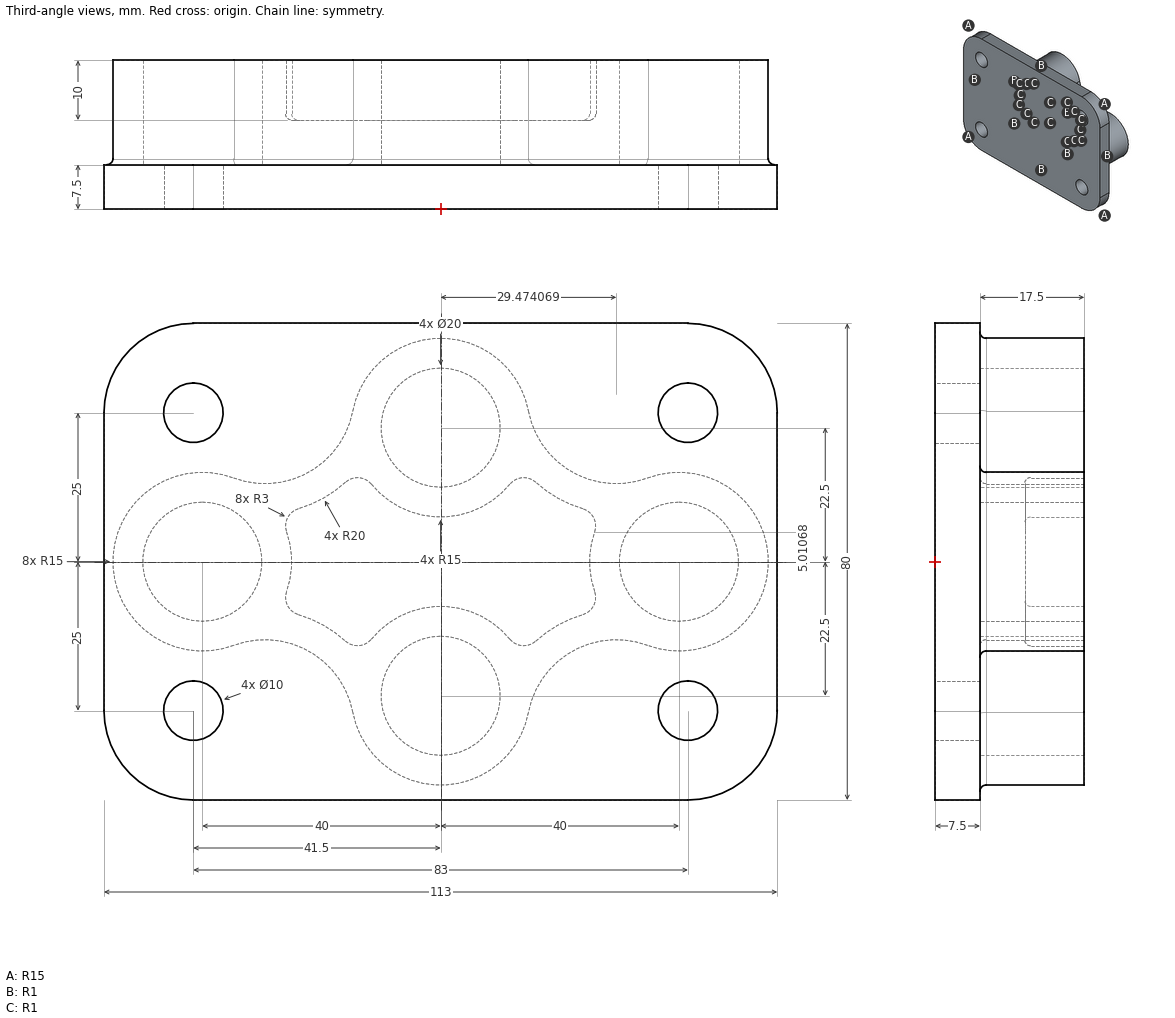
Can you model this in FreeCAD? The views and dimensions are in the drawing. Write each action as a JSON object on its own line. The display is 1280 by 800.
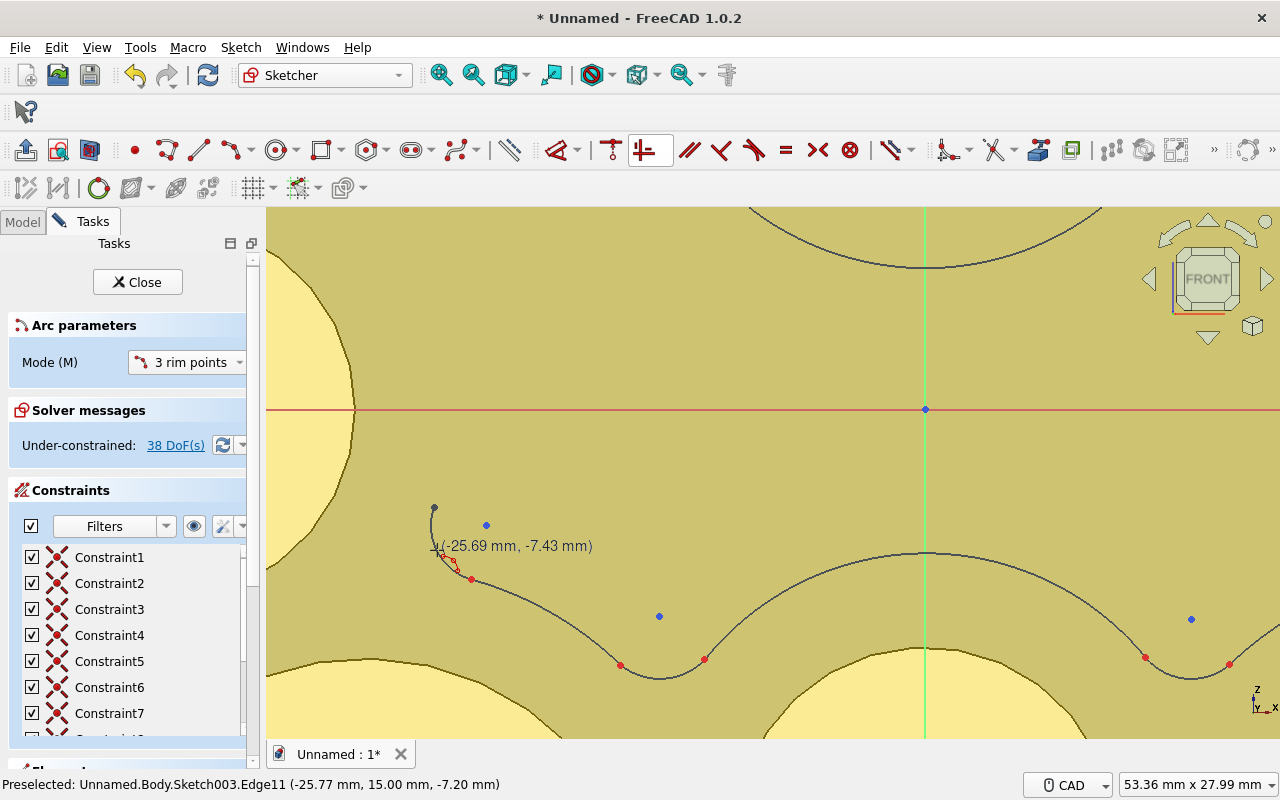
{"action": "left_click", "coordinate": [434, 508]}
{"action": "left_click", "coordinate": [434, 315]}
{"action": "left_click", "coordinate": [449, 429]}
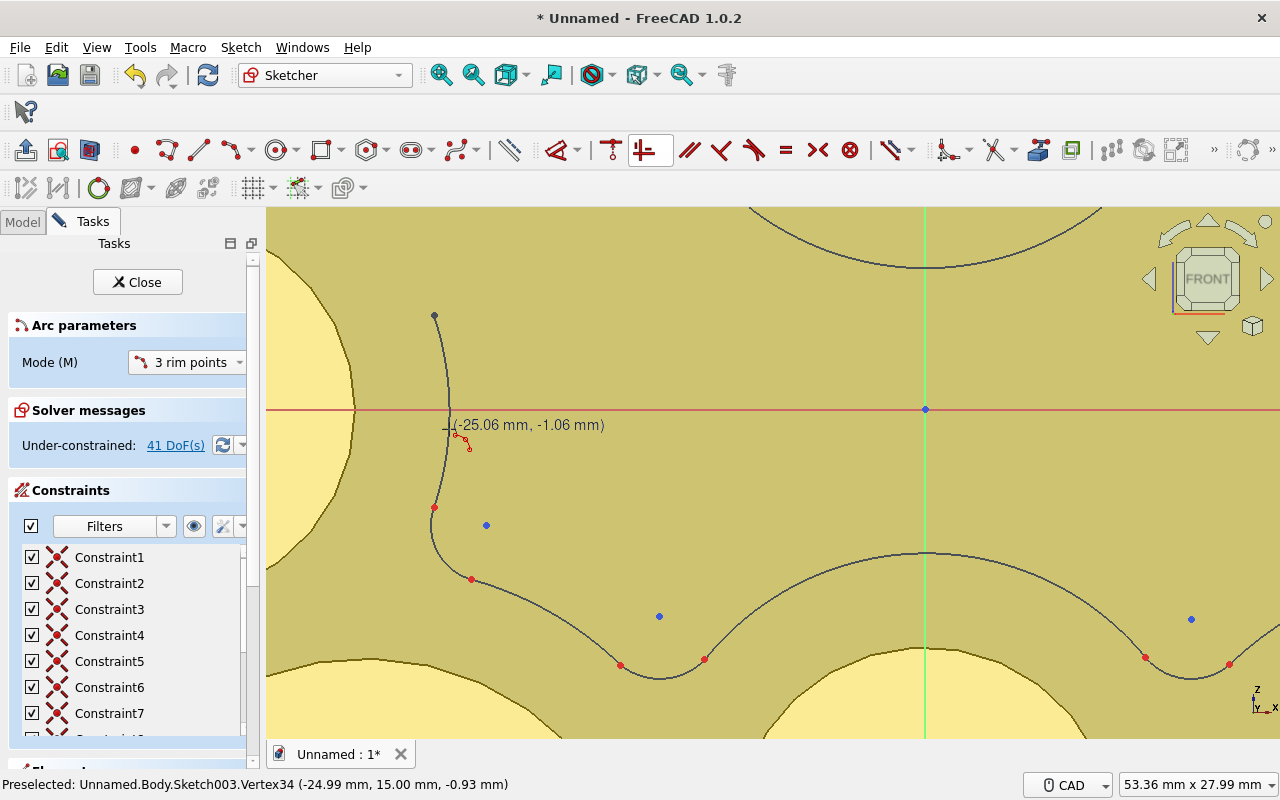
{"action": "left_click", "coordinate": [434, 316]}
{"action": "left_click", "coordinate": [471, 241]}
{"action": "left_click", "coordinate": [437, 270]}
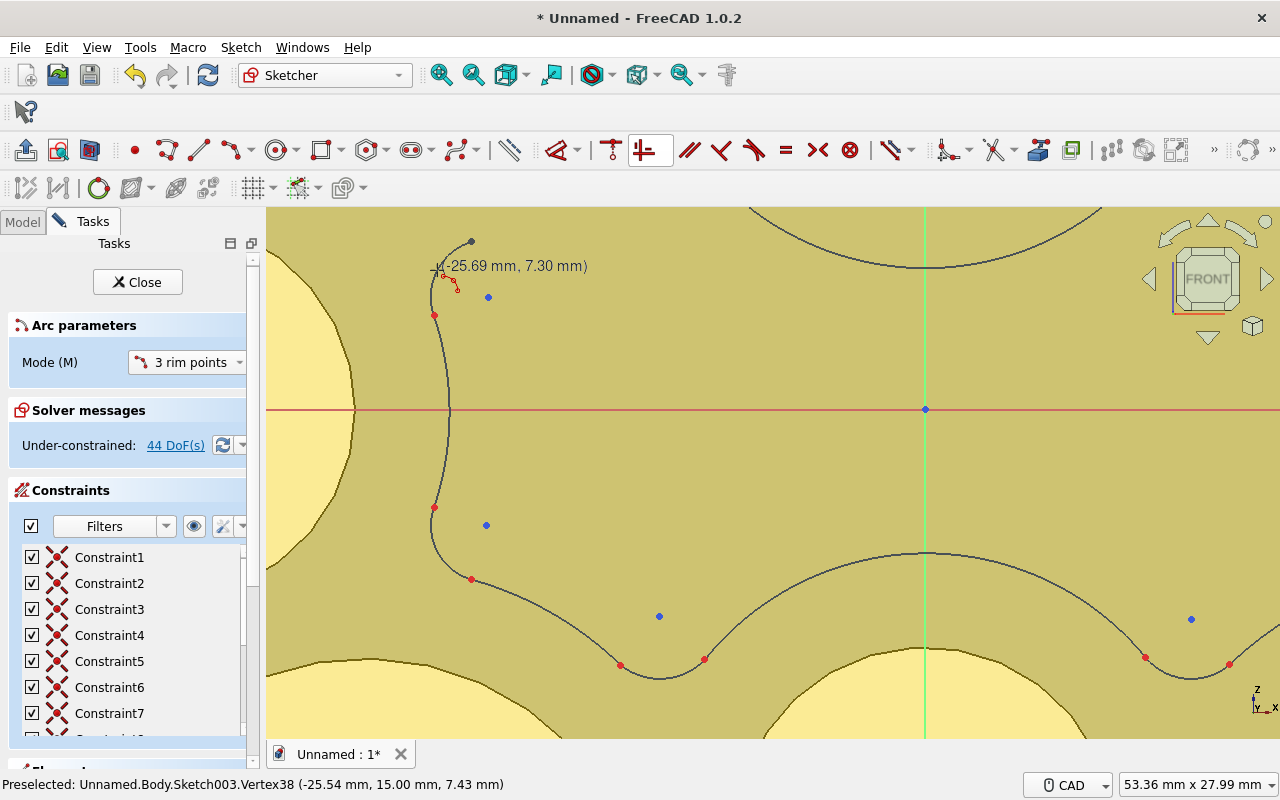
{"action": "left_click", "coordinate": [471, 242]}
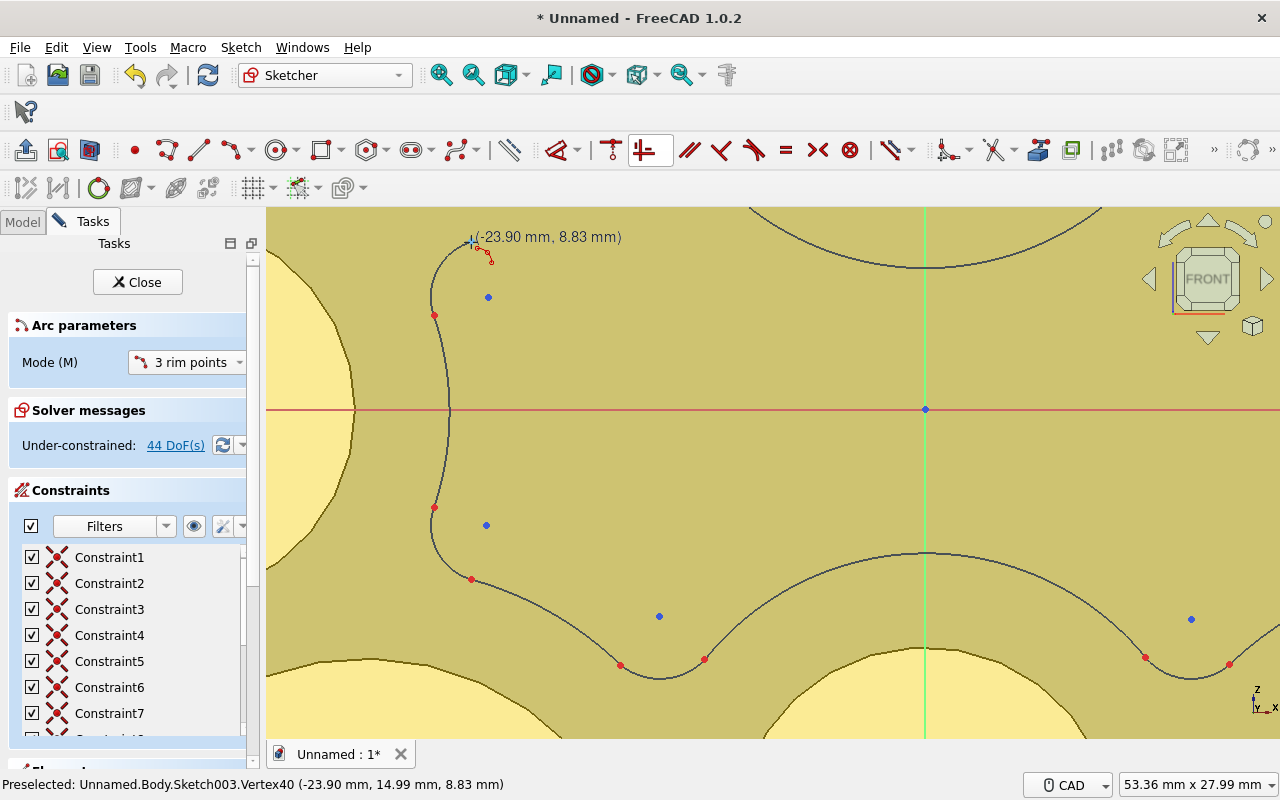
{"action": "scroll", "coordinate": [436, 550], "scroll_direction": "down", "scroll_amount": 3}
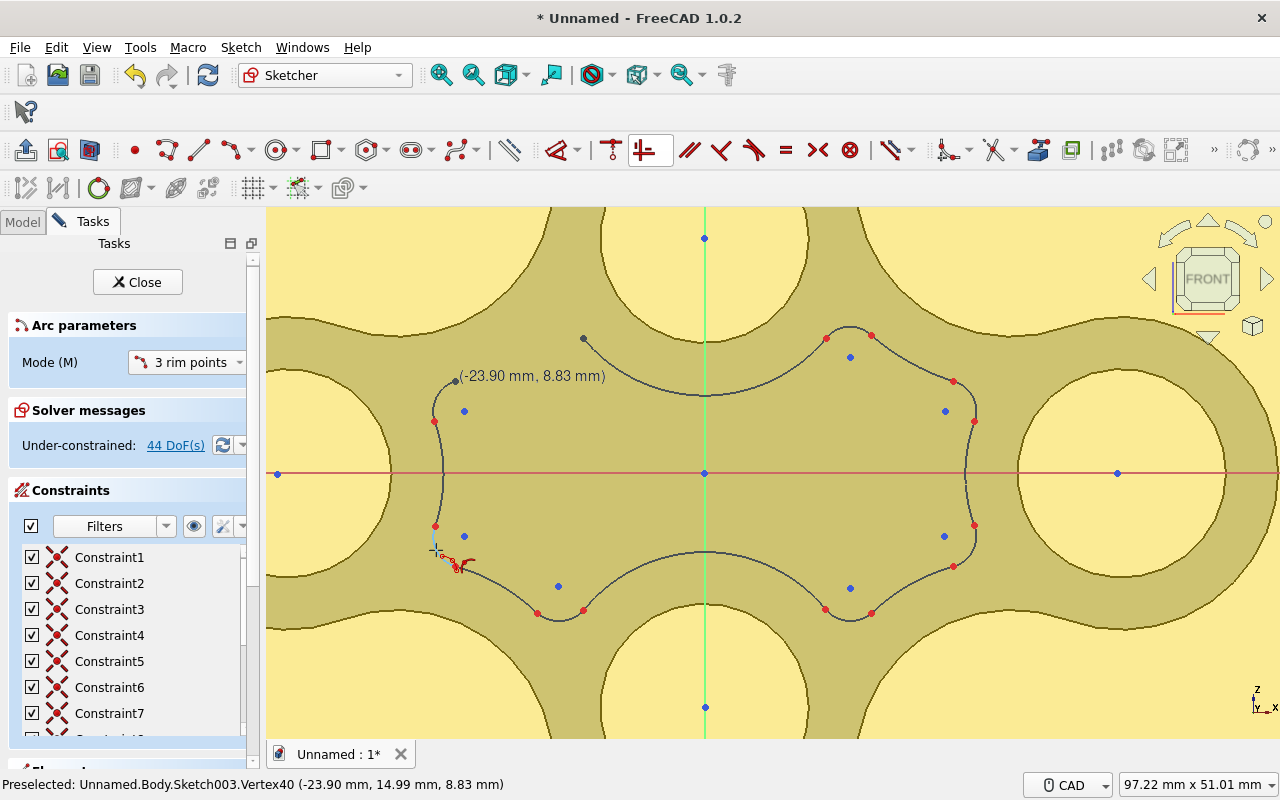
{"action": "left_click", "coordinate": [538, 334]}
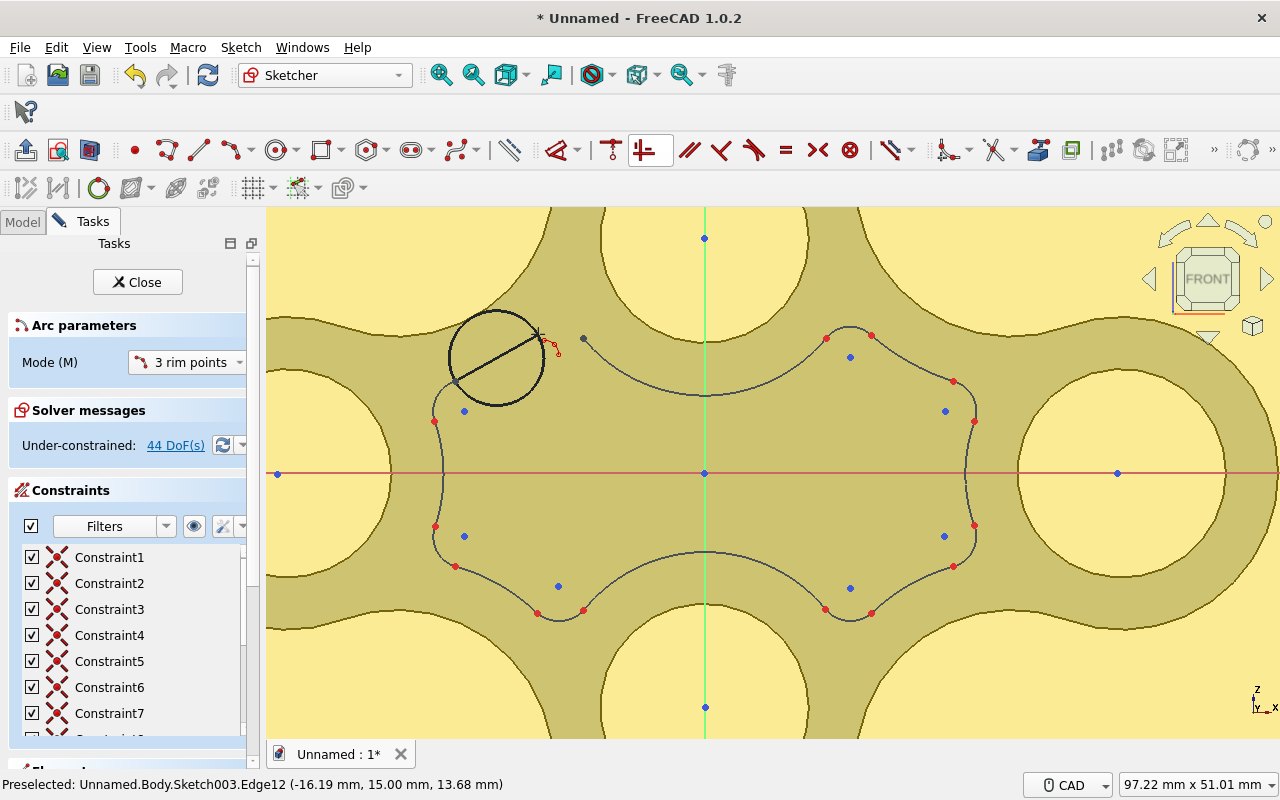
{"action": "scroll", "coordinate": [499, 362], "scroll_direction": "up", "scroll_amount": 6}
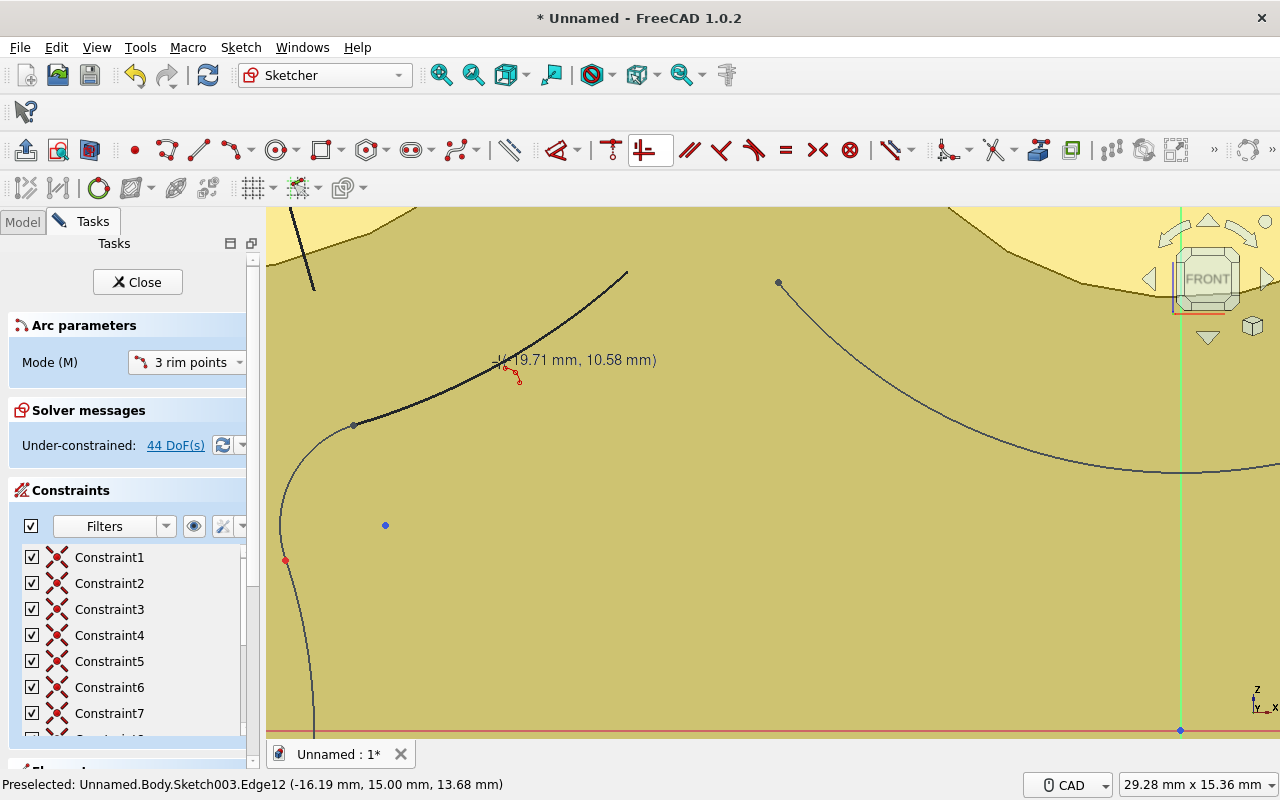
{"action": "left_click", "coordinate": [500, 362]}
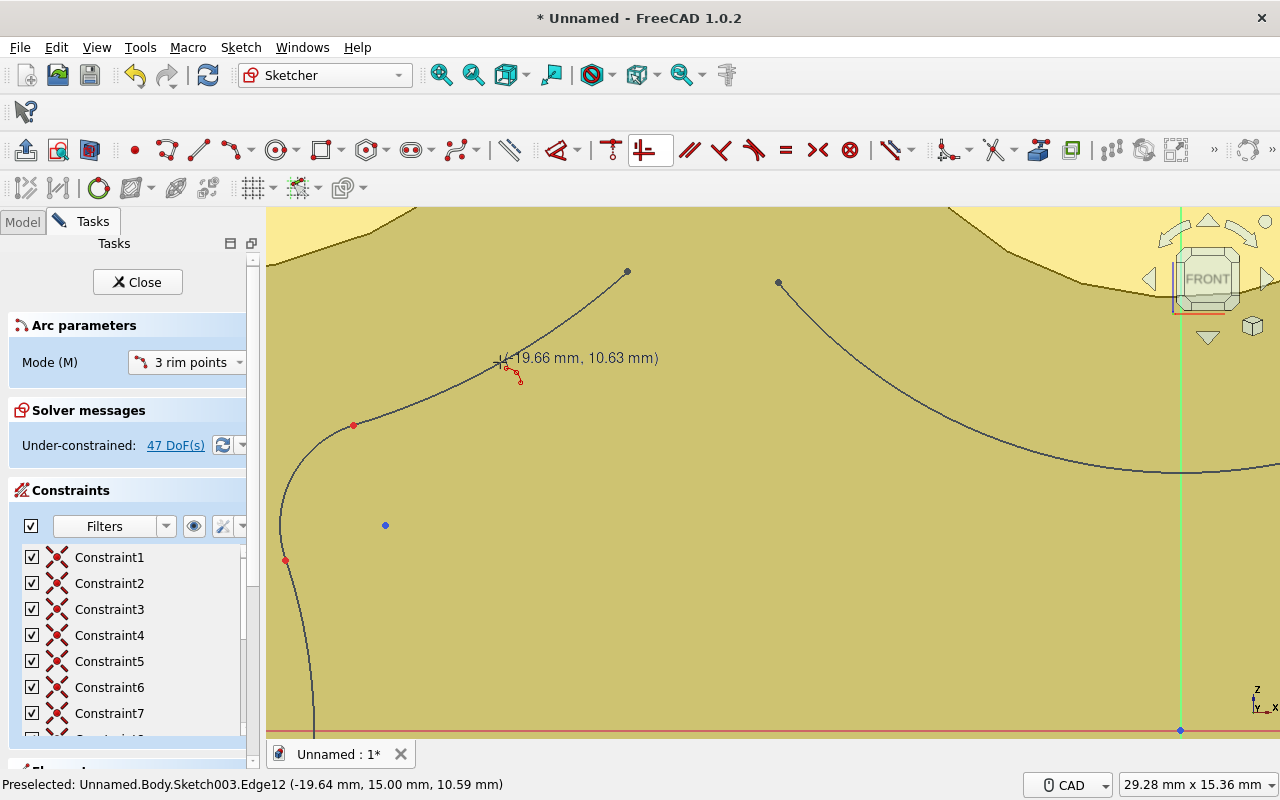
{"action": "left_click", "coordinate": [628, 272]}
{"action": "left_click", "coordinate": [778, 282]}
{"action": "left_click", "coordinate": [705, 242]}
{"action": "key", "text": "Escape"}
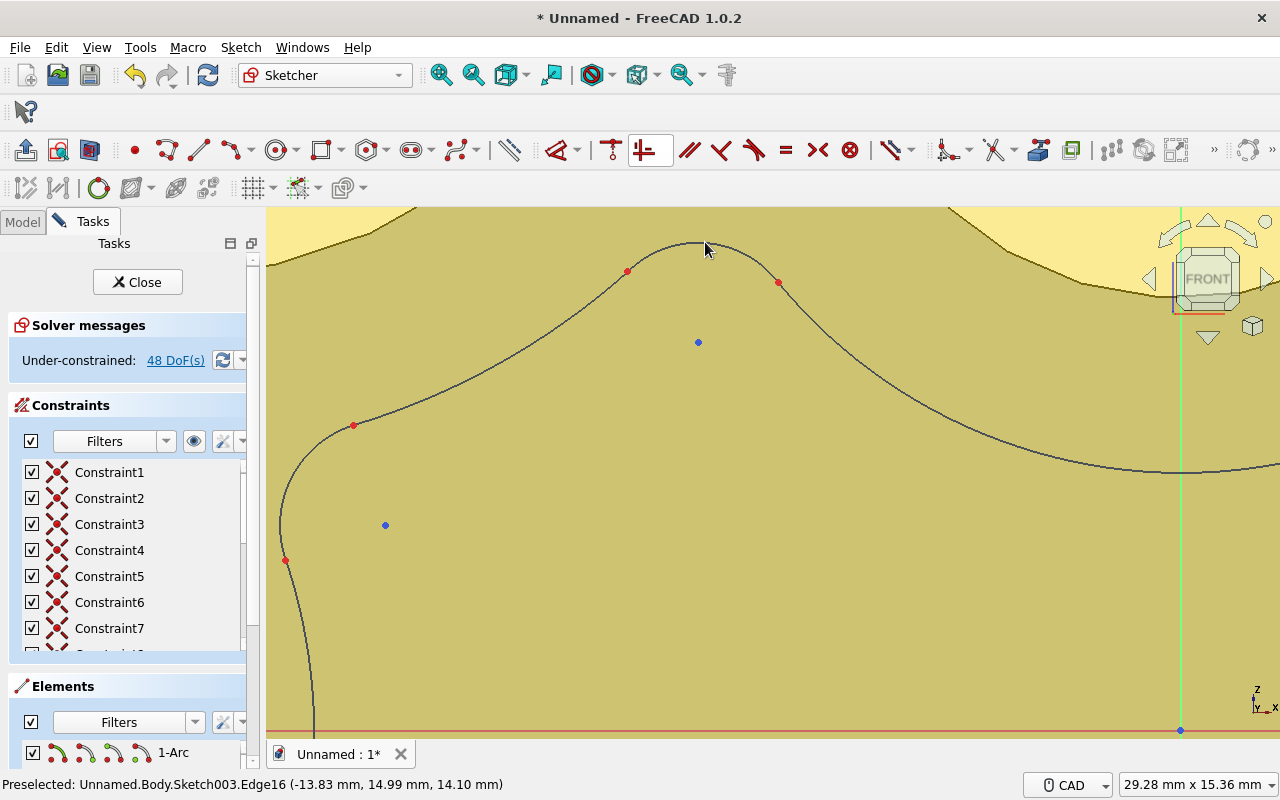
{"action": "left_click", "coordinate": [1001, 441]}